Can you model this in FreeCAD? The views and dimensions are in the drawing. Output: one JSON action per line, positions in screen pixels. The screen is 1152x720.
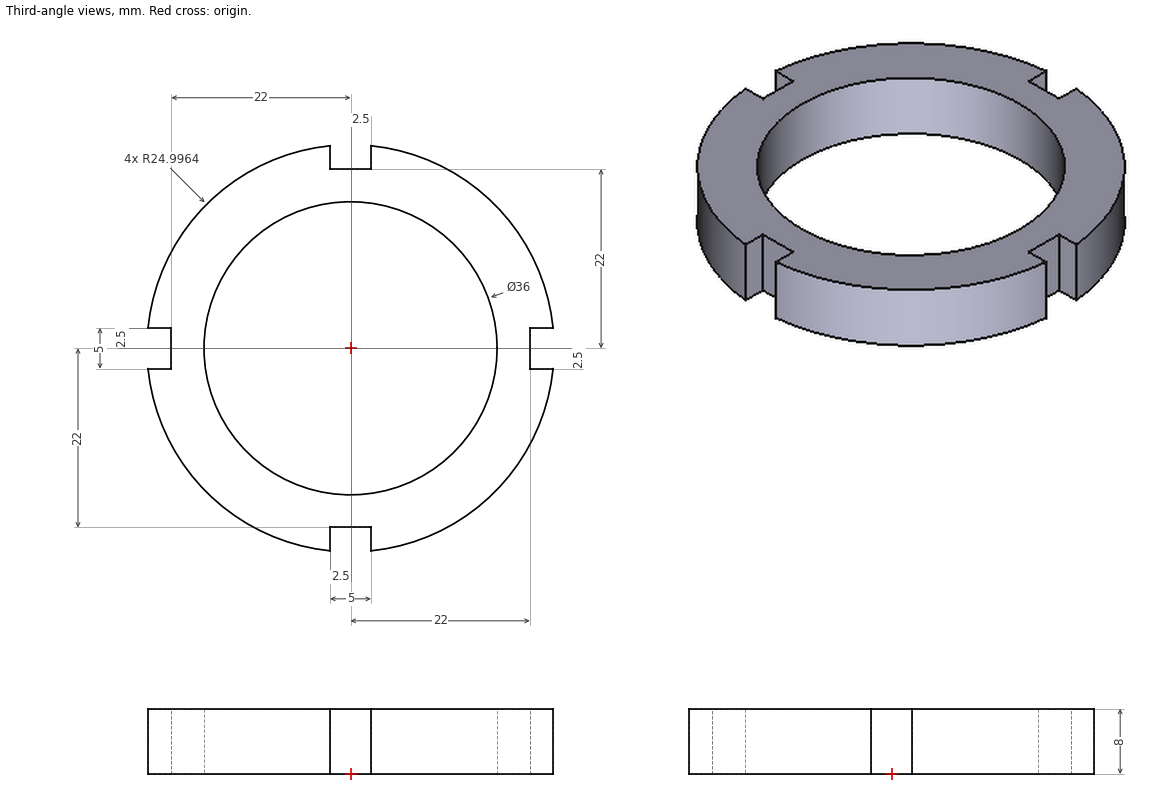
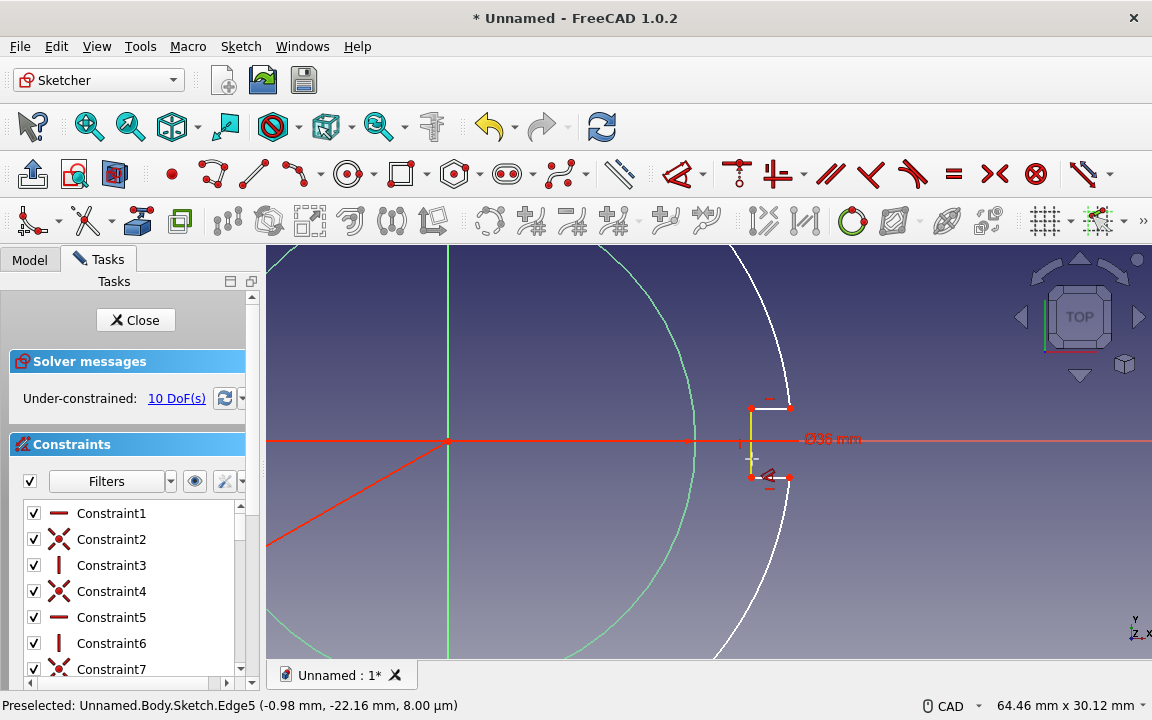
{"action": "left_click", "coordinate": [751, 457]}
{"action": "left_click", "coordinate": [785, 427]}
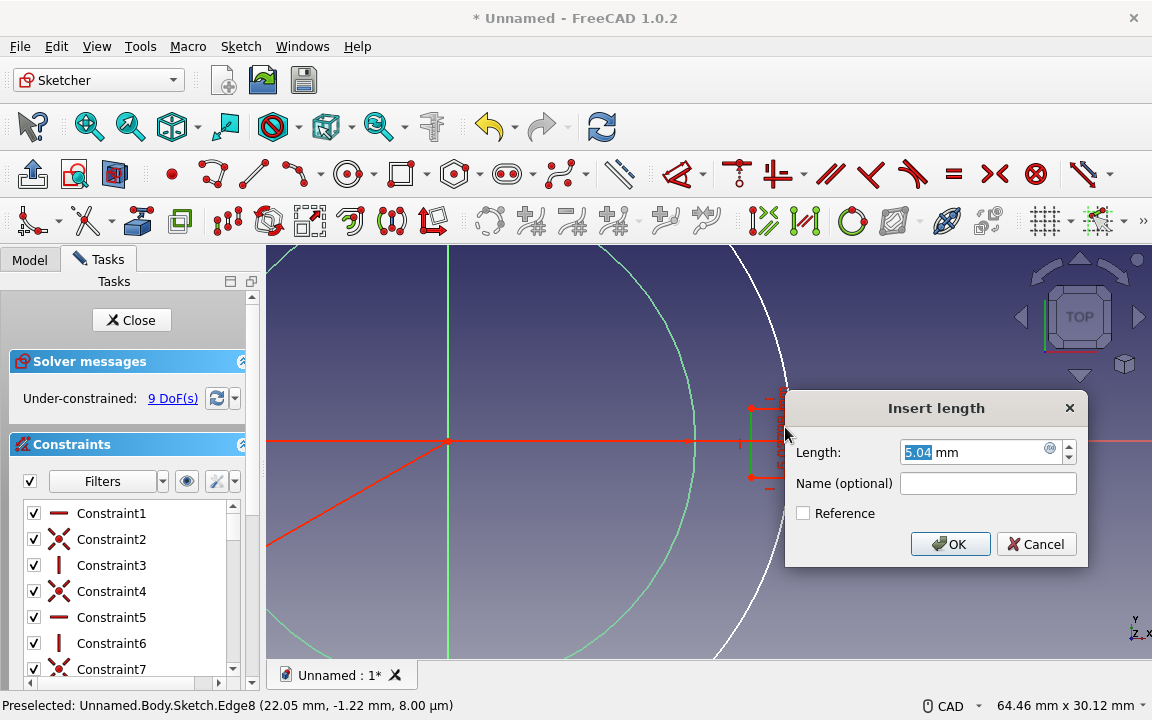
{"action": "type", "text": "5"}
{"action": "key", "text": "Return"}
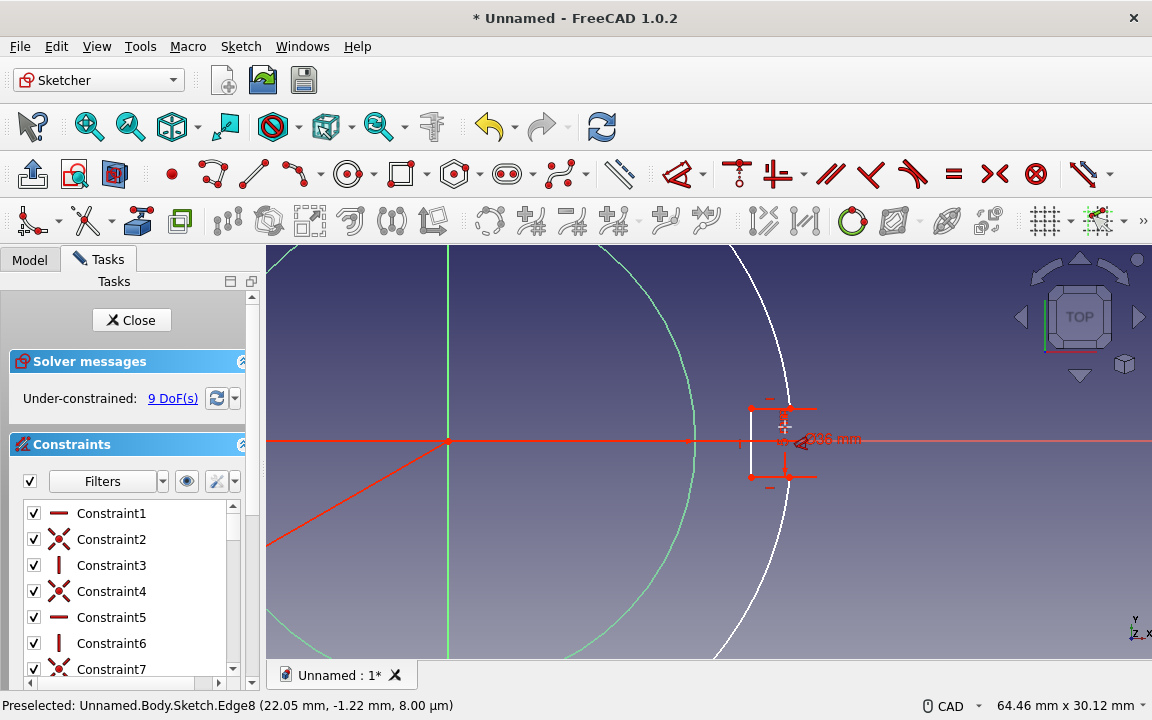
{"action": "scroll", "coordinate": [752, 458], "scroll_direction": "down", "scroll_amount": 5}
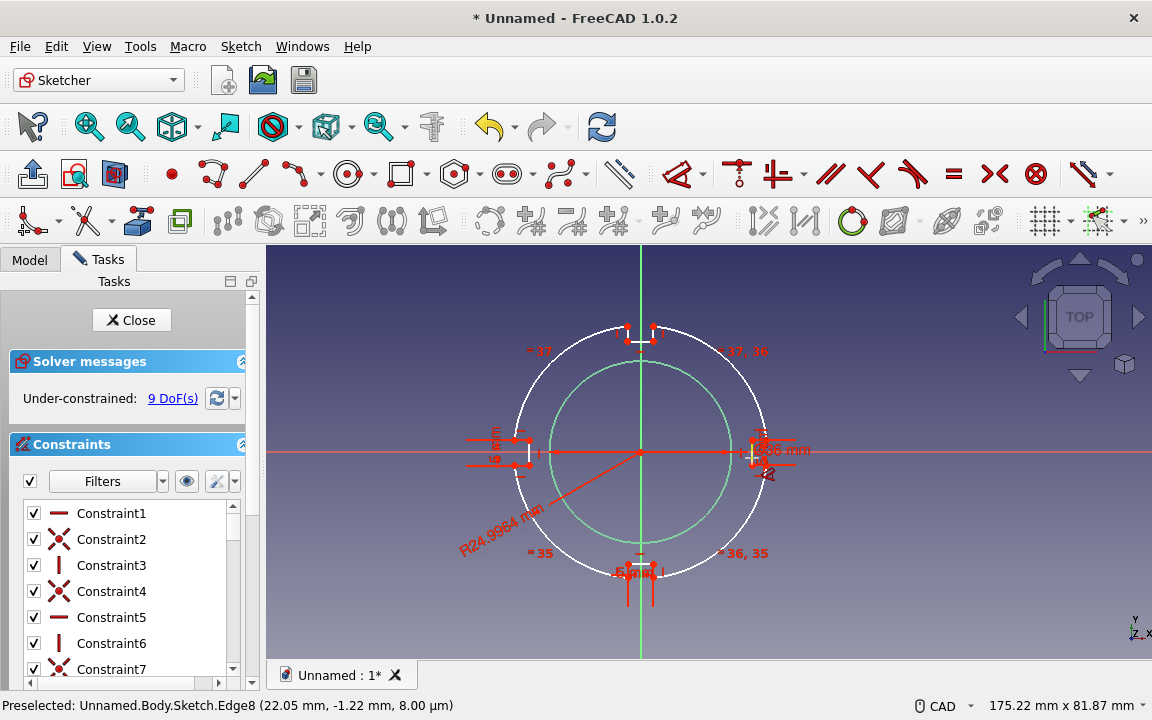
{"action": "scroll", "coordinate": [645, 342], "scroll_direction": "up", "scroll_amount": 6}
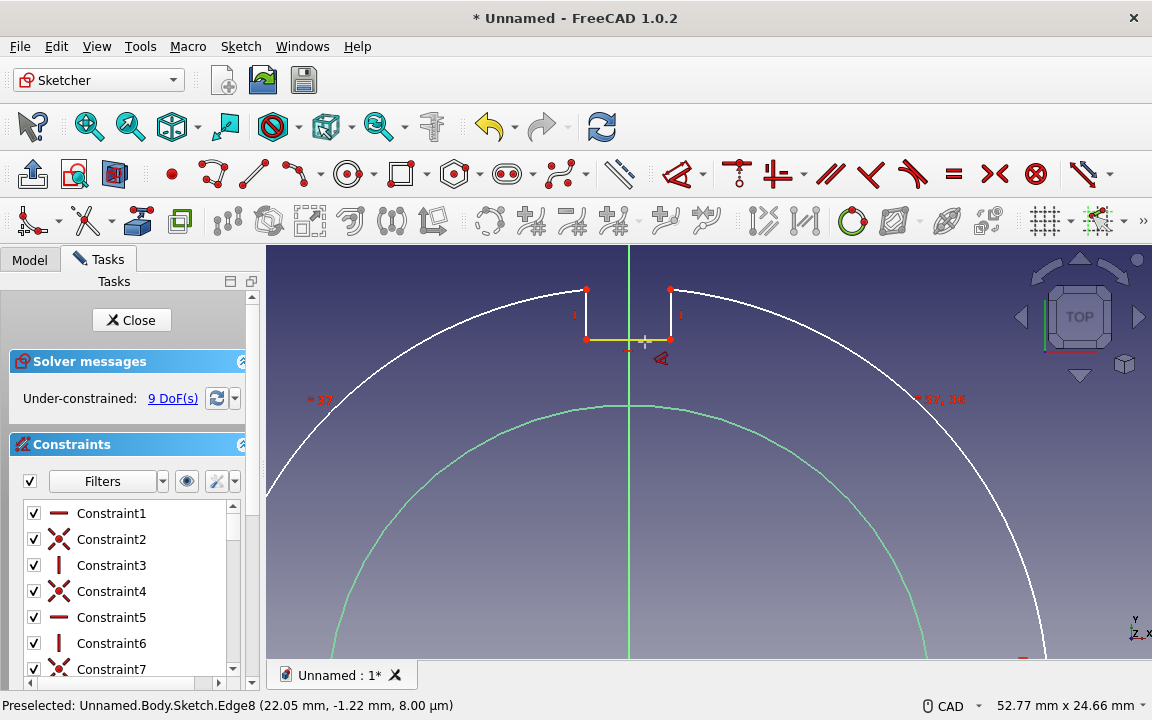
{"action": "left_click", "coordinate": [645, 340]}
{"action": "left_click", "coordinate": [609, 306]}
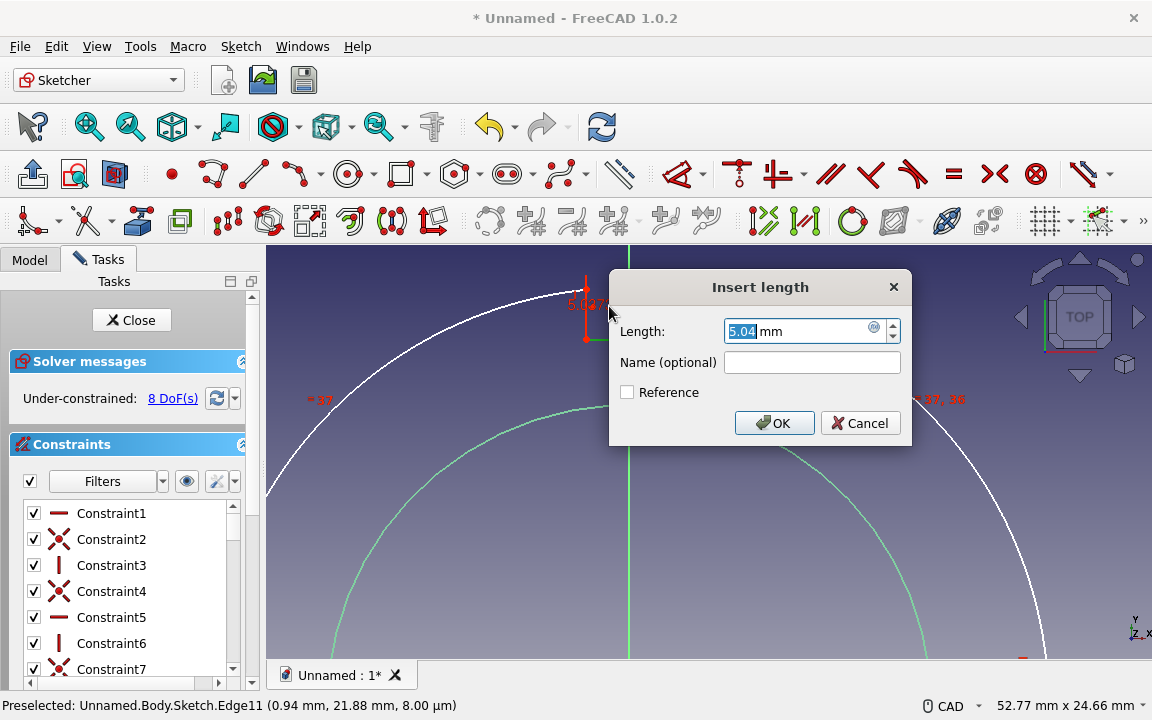
{"action": "type", "text": "5"}
{"action": "key", "text": "Return"}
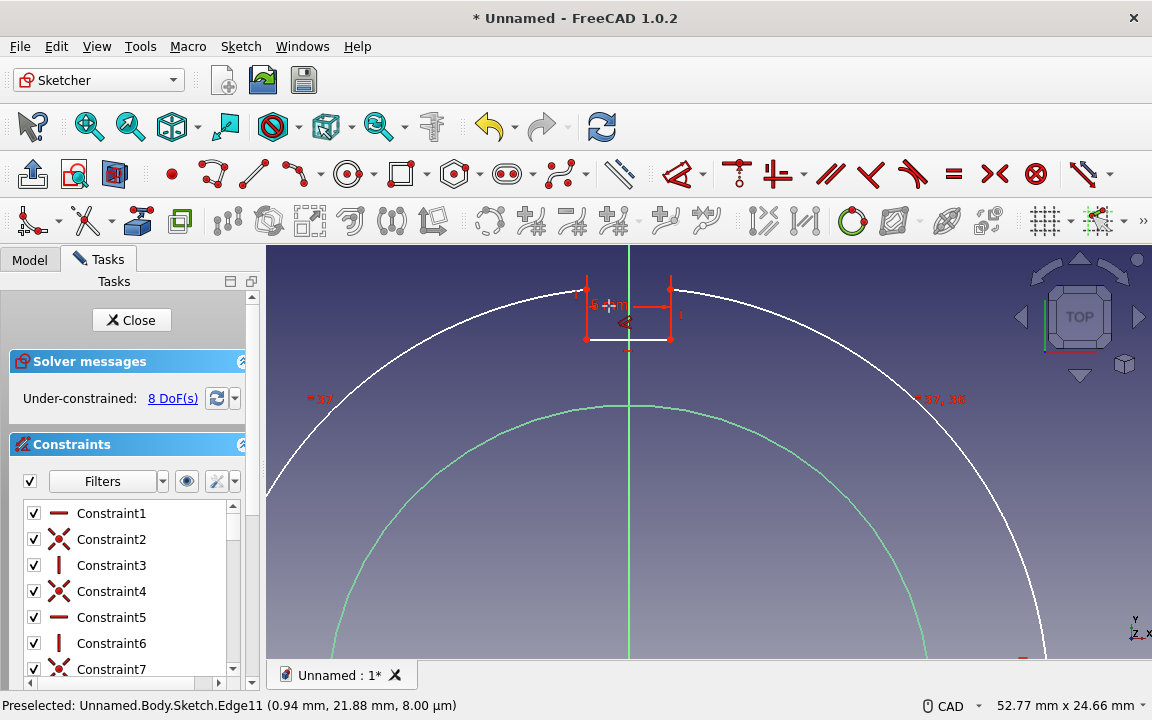
{"action": "scroll", "coordinate": [645, 342], "scroll_direction": "down", "scroll_amount": 6}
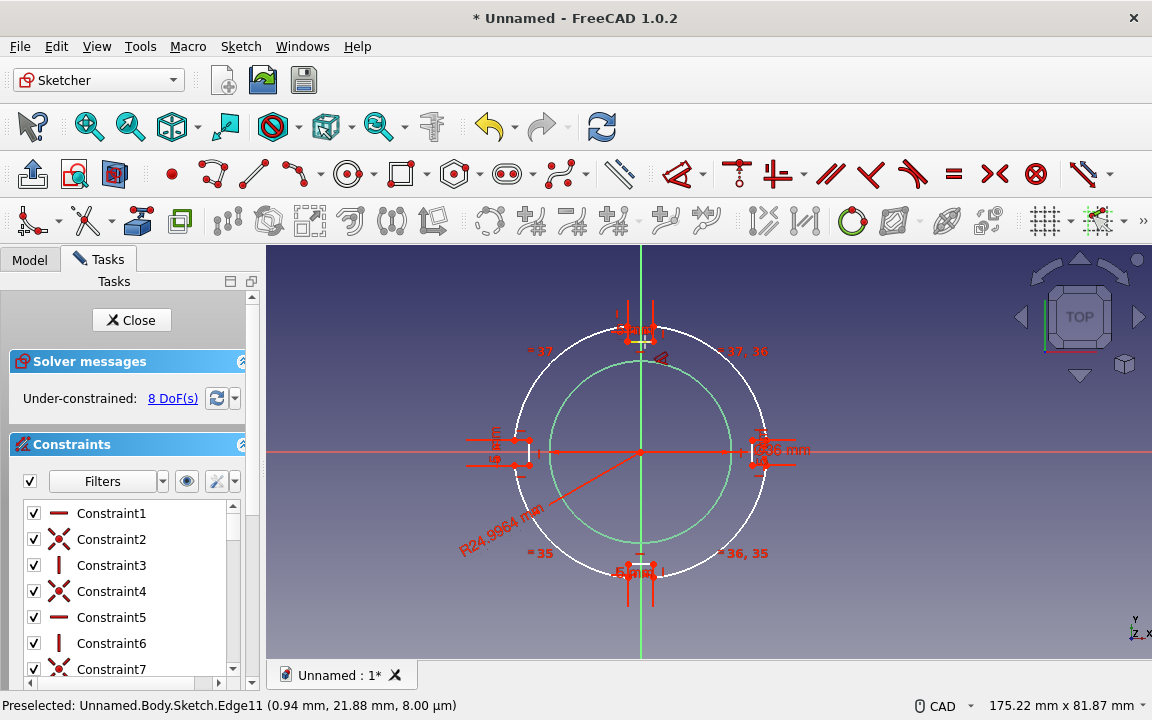
{"action": "left_click", "coordinate": [529, 440]}
{"action": "left_click", "coordinate": [585, 406]}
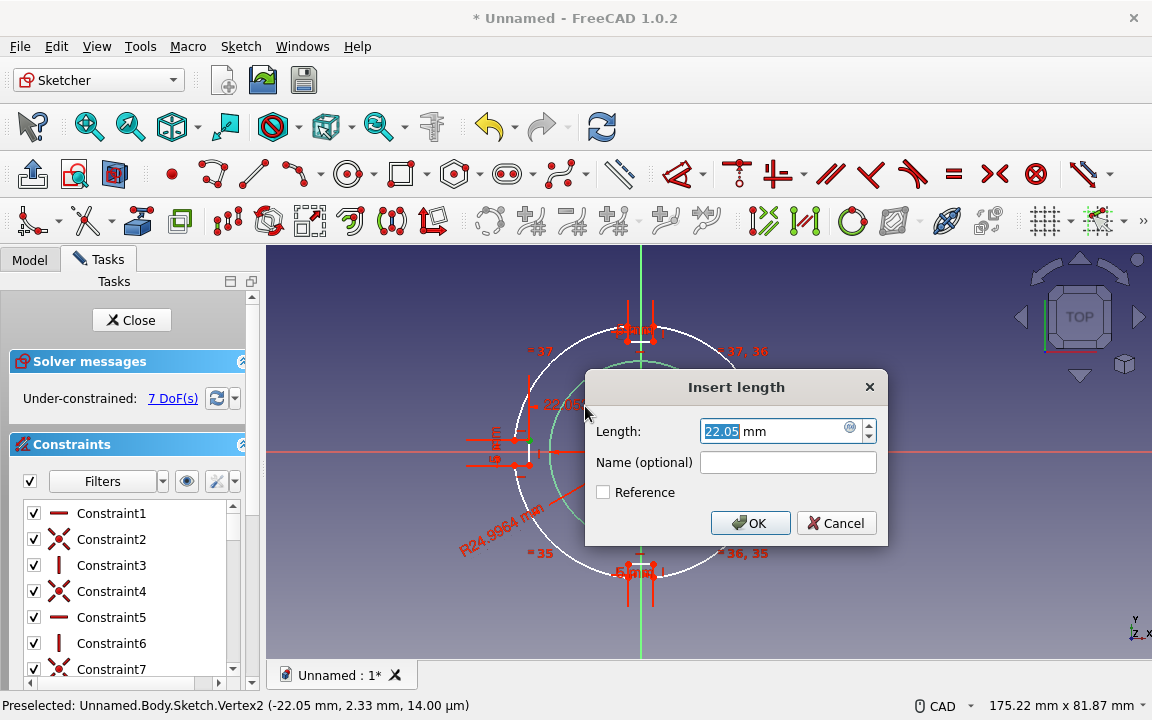
{"action": "type", "text": "22"}
{"action": "key", "text": "Return"}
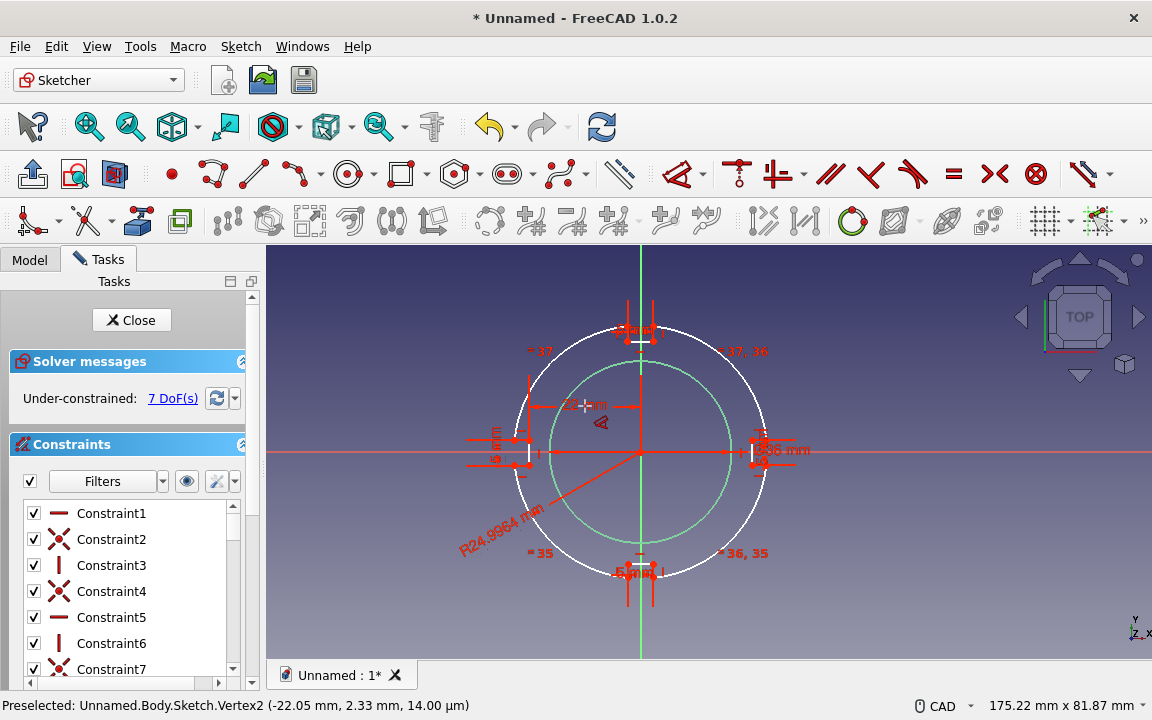
{"action": "left_click", "coordinate": [628, 564]}
{"action": "left_click", "coordinate": [594, 508]}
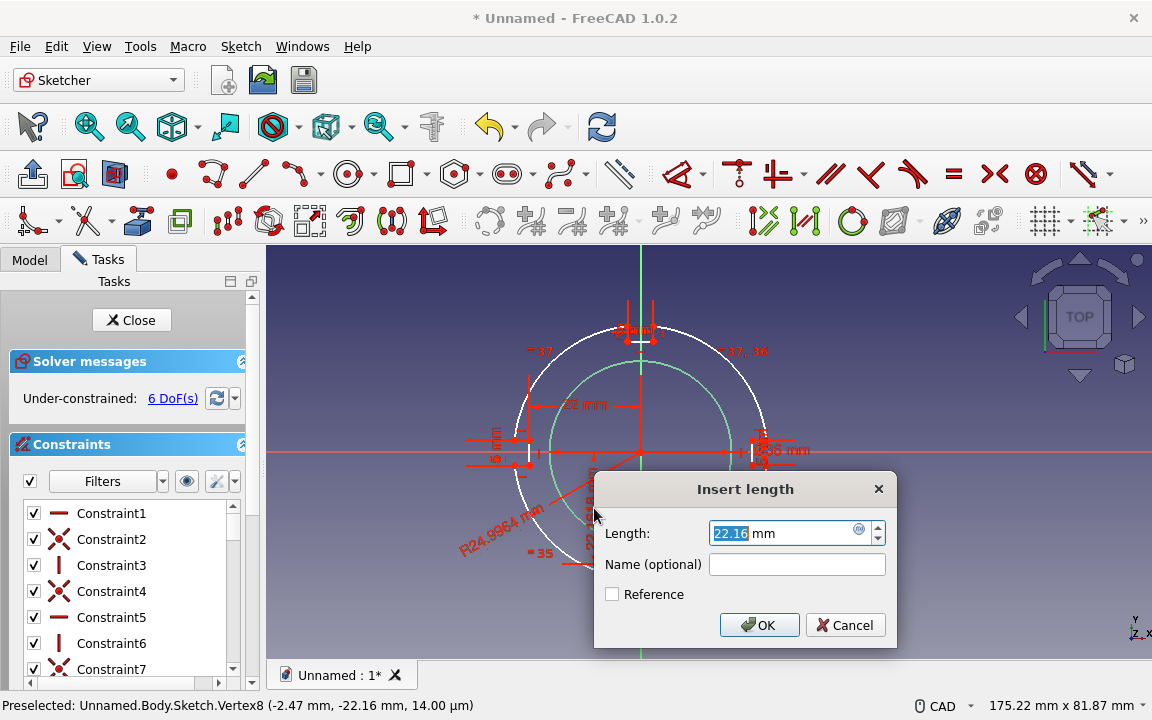
{"action": "type", "text": "22"}
{"action": "key", "text": "Return"}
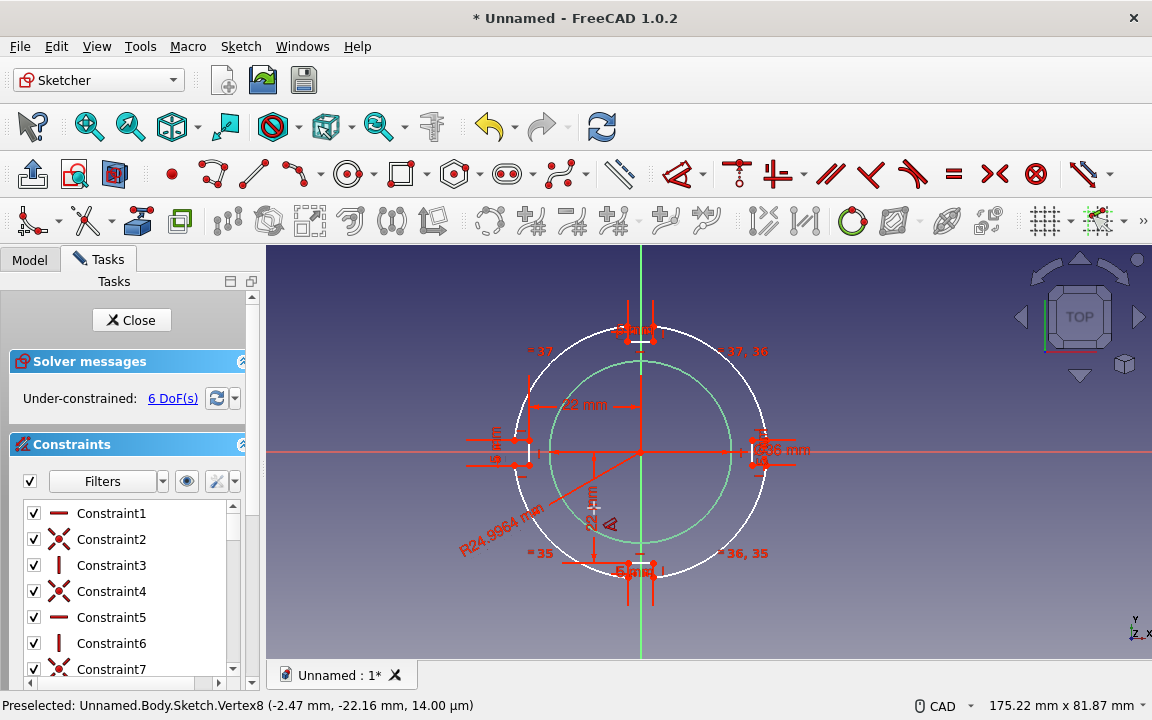
{"action": "left_click", "coordinate": [752, 465]}
{"action": "left_click", "coordinate": [696, 499]}